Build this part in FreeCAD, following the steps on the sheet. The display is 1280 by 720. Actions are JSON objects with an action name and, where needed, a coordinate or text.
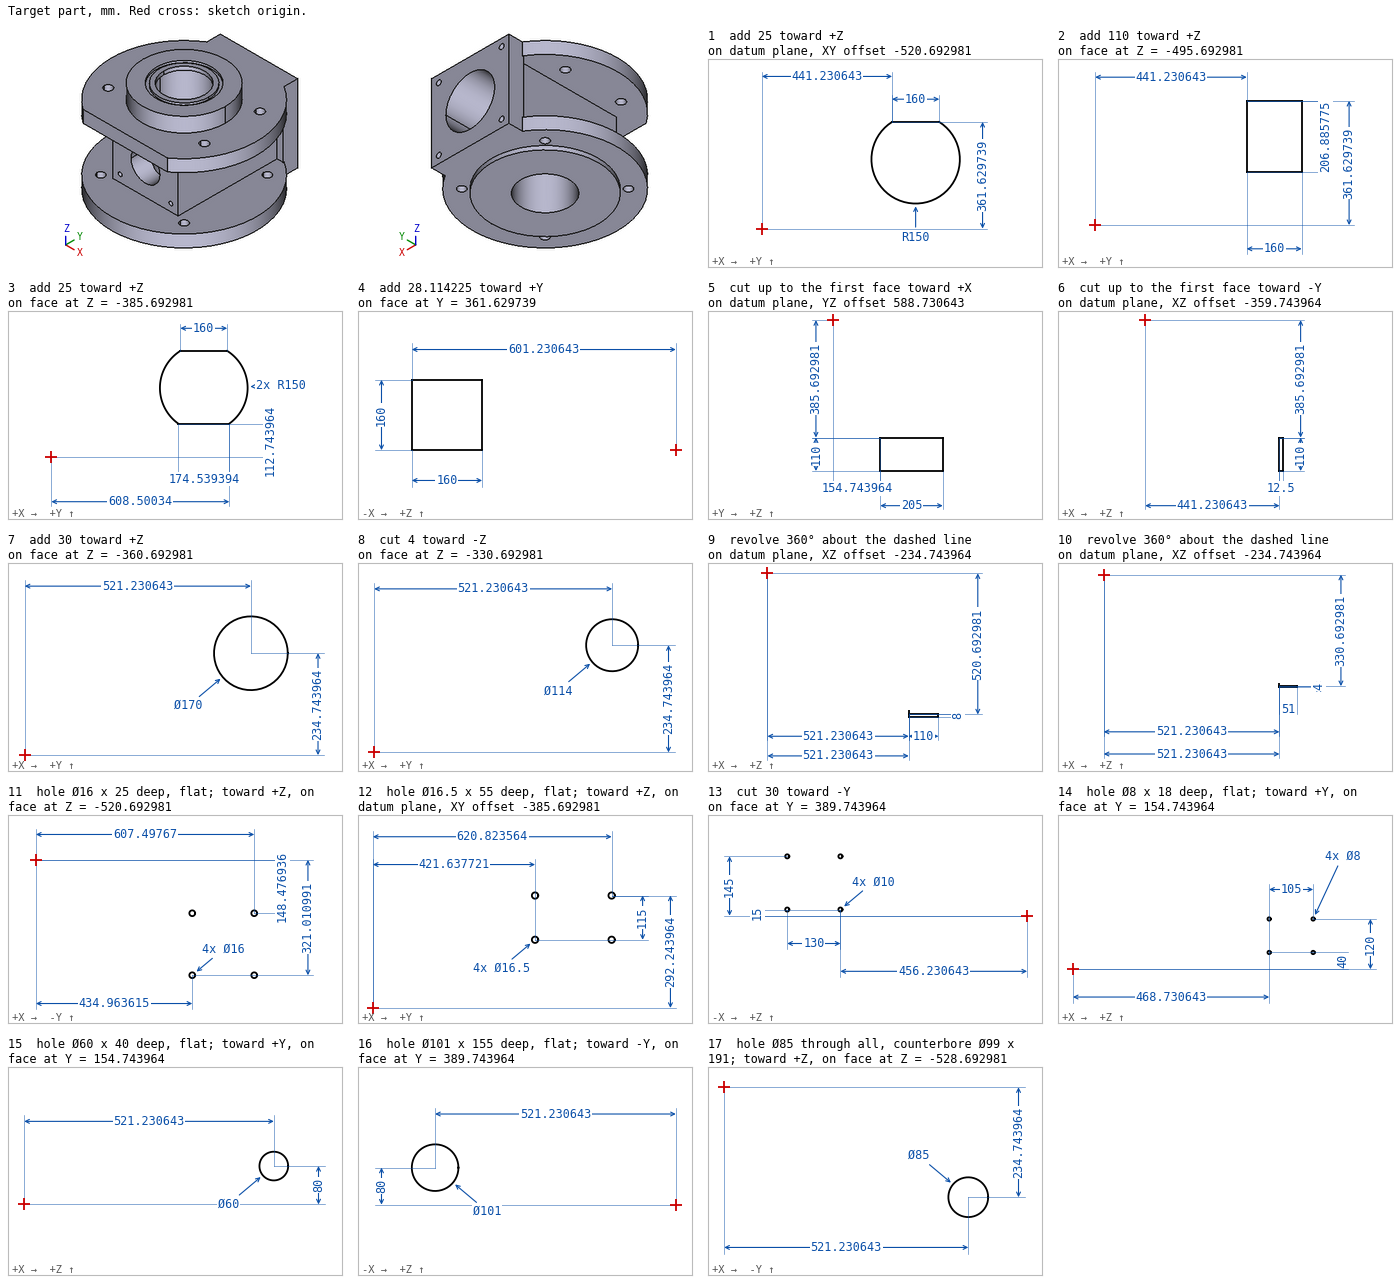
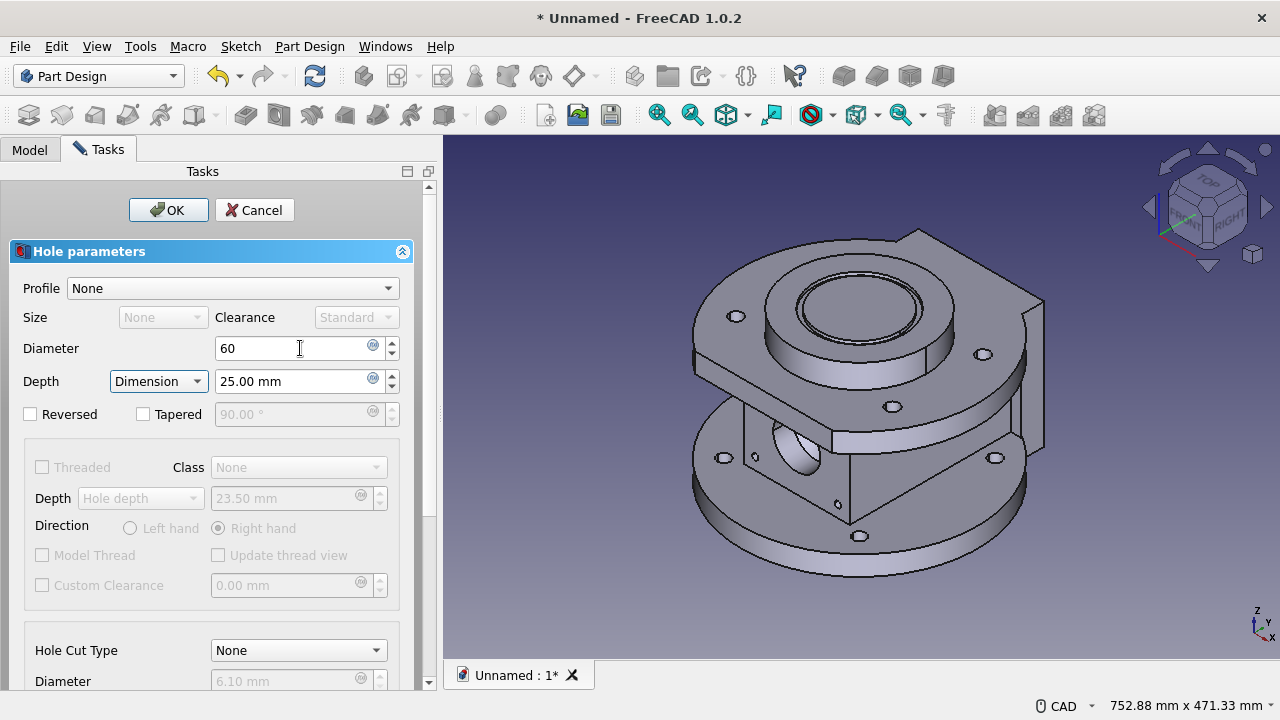
{"action": "triple_click", "coordinate": [300, 382]}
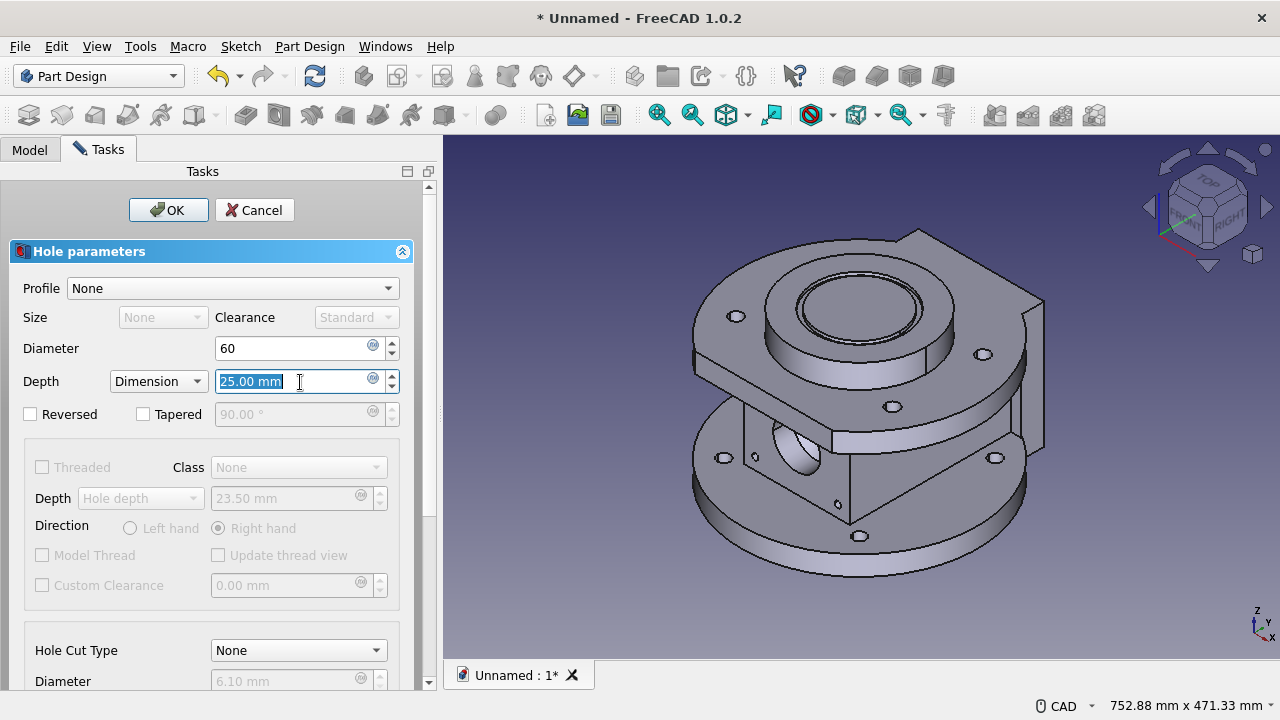
{"action": "type", "text": "40"}
{"action": "key", "text": "Tab"}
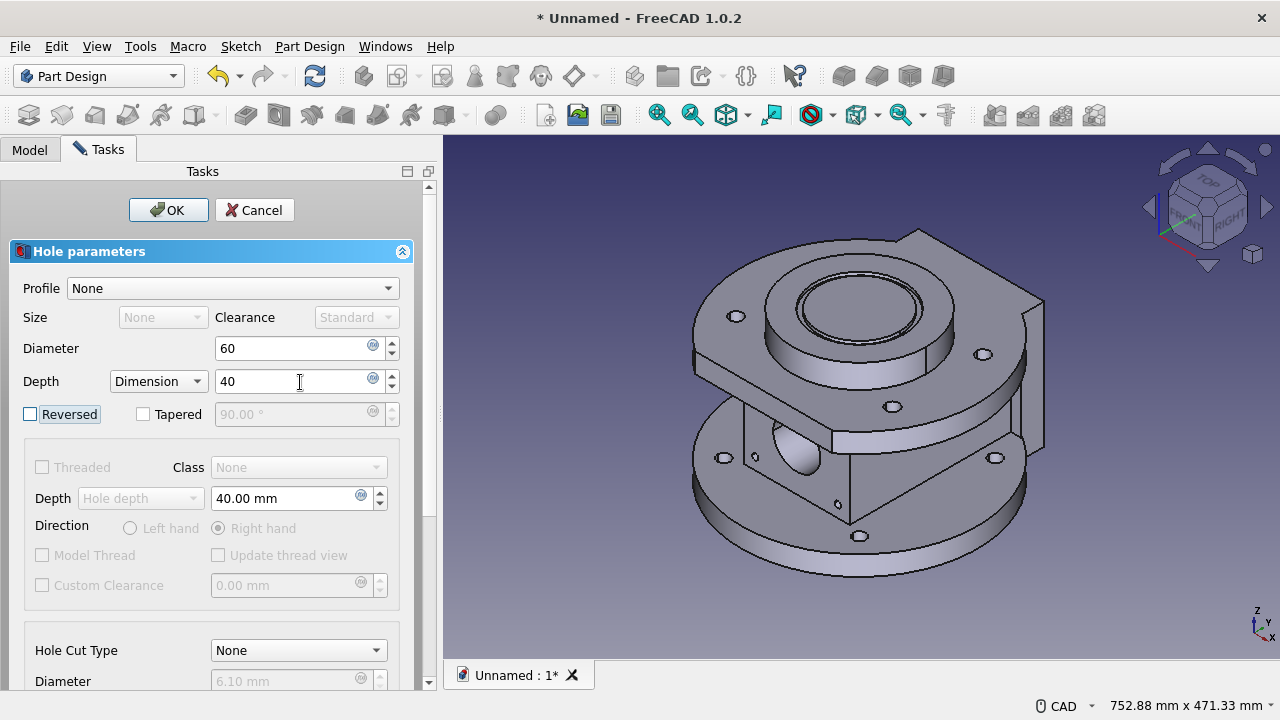
{"action": "scroll", "coordinate": [429, 436], "scroll_direction": "down", "scroll_amount": 4}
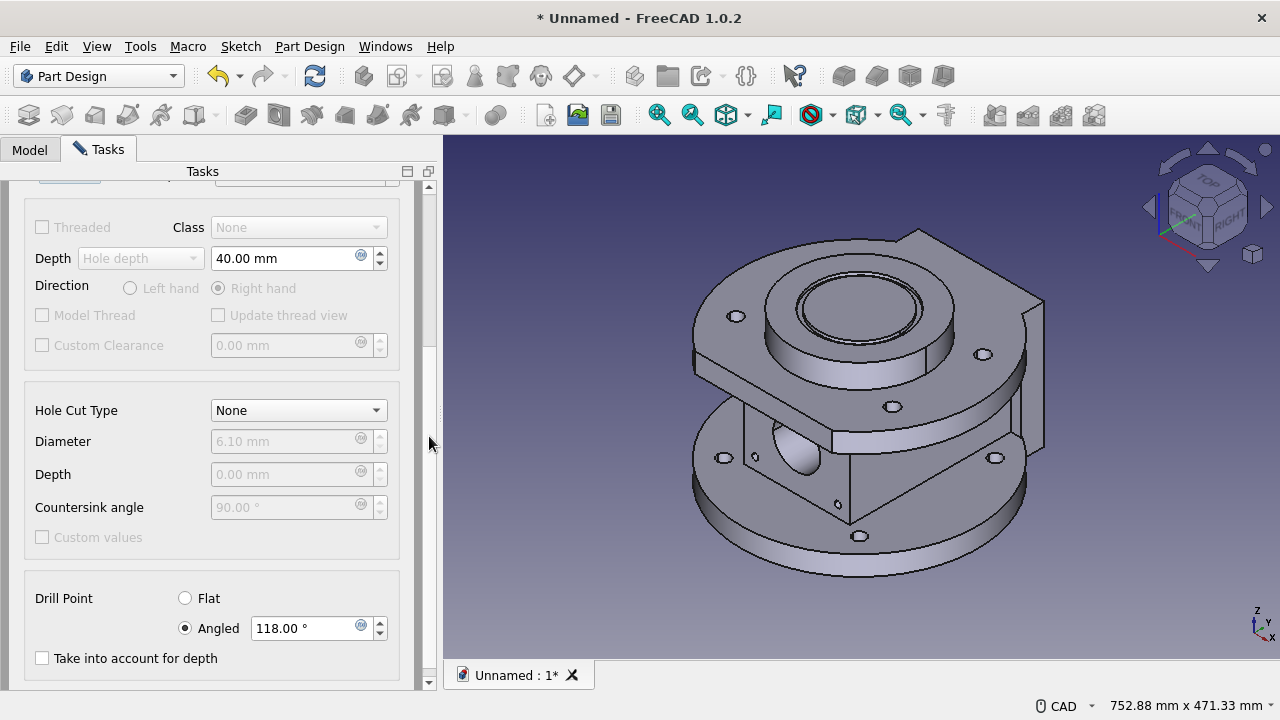
{"action": "left_click", "coordinate": [186, 596]}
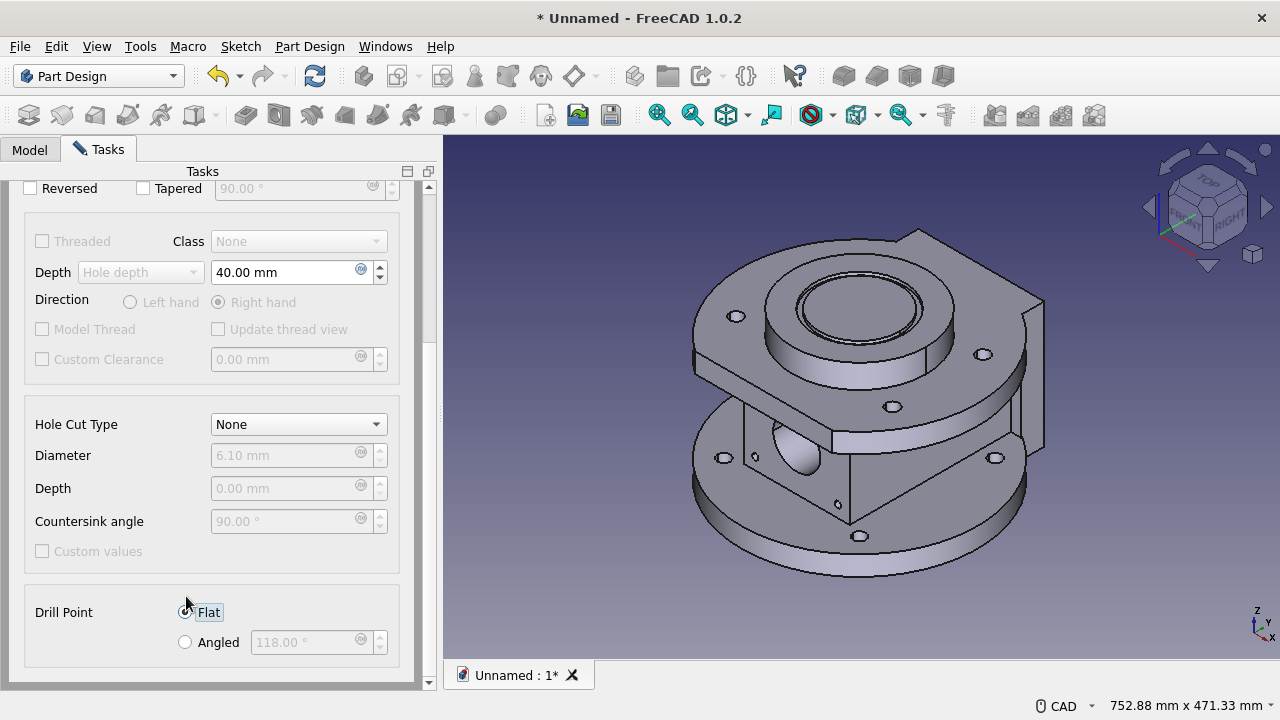
{"action": "scroll", "coordinate": [429, 436], "scroll_direction": "up", "scroll_amount": 5}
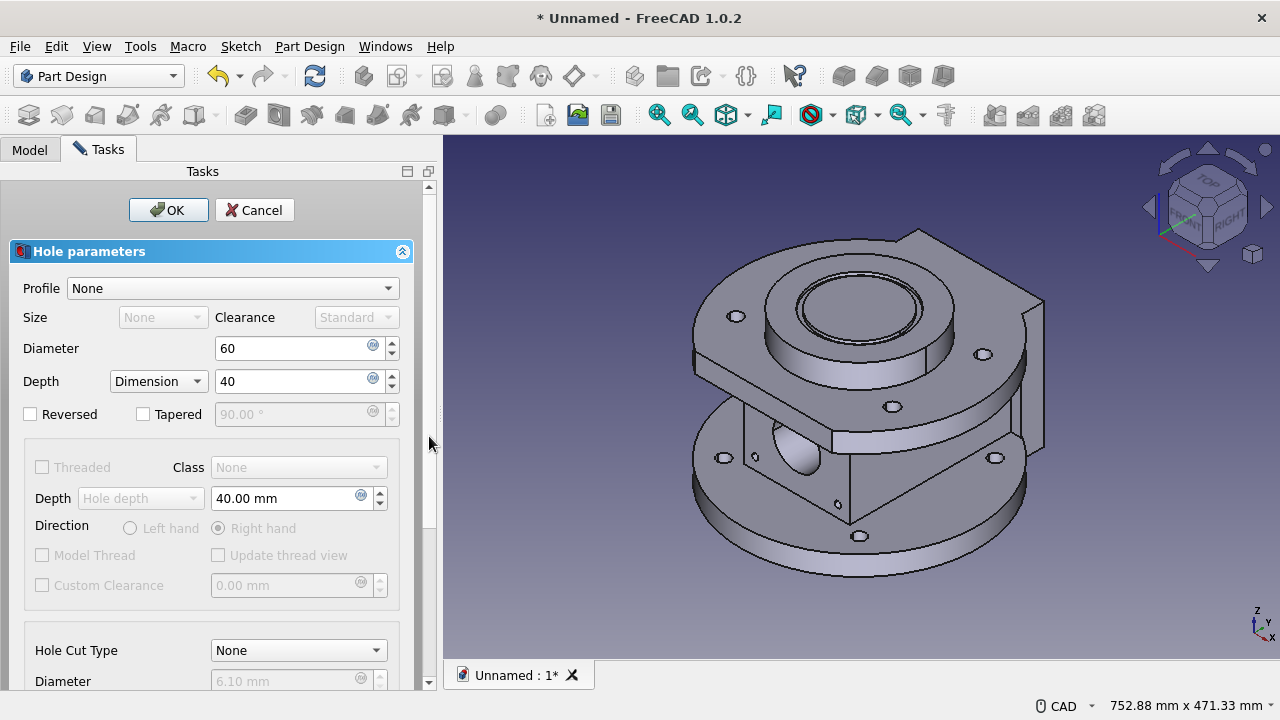
{"action": "left_click", "coordinate": [169, 210]}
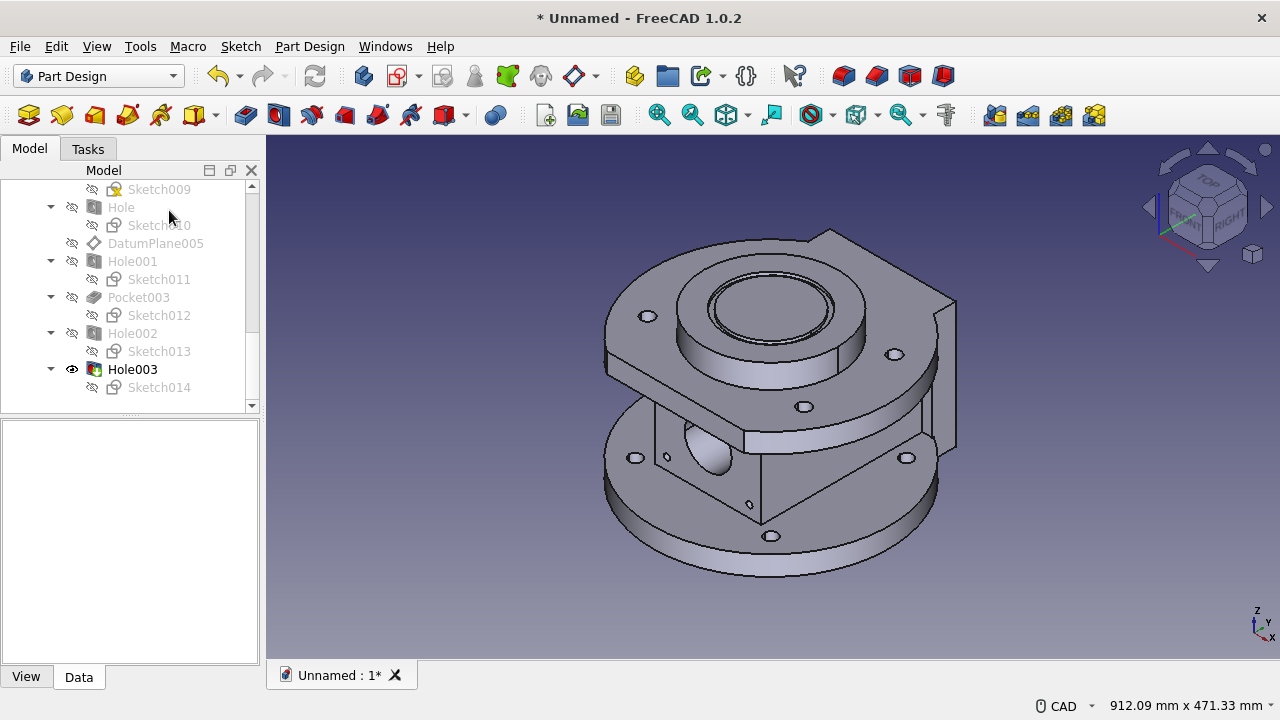
{"action": "key", "text": "4"}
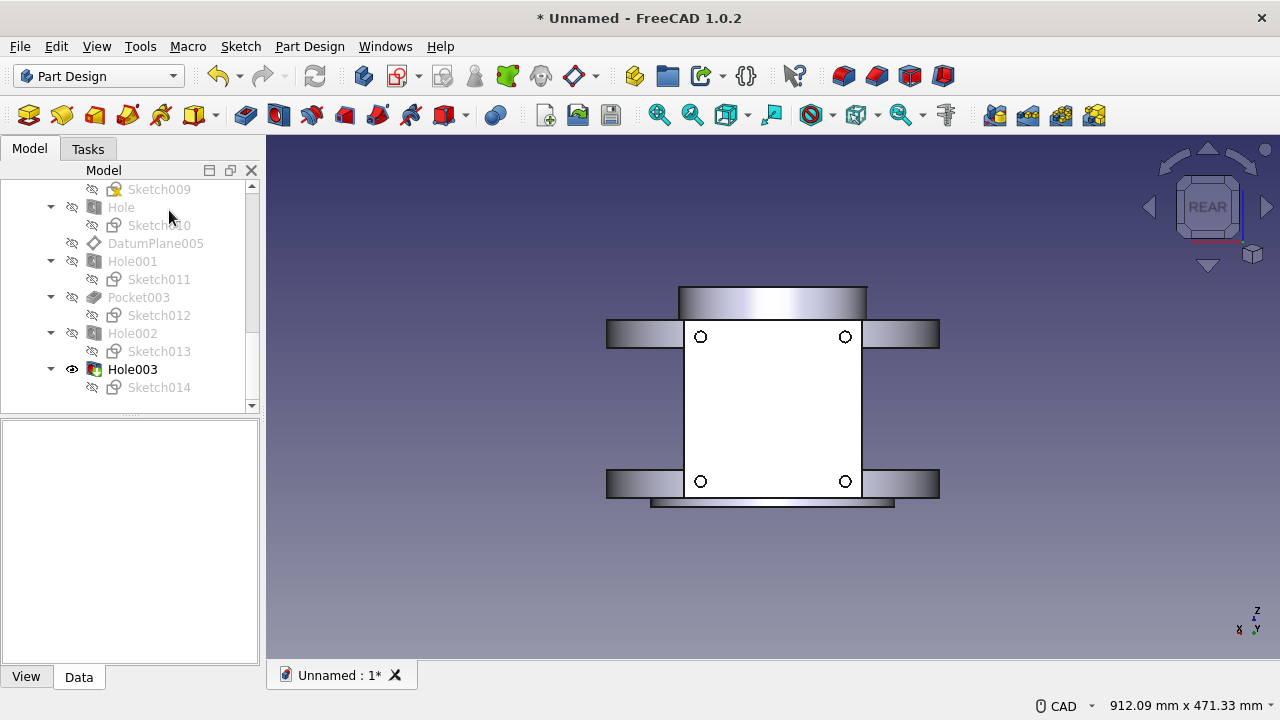
{"action": "left_click", "coordinate": [660, 116]}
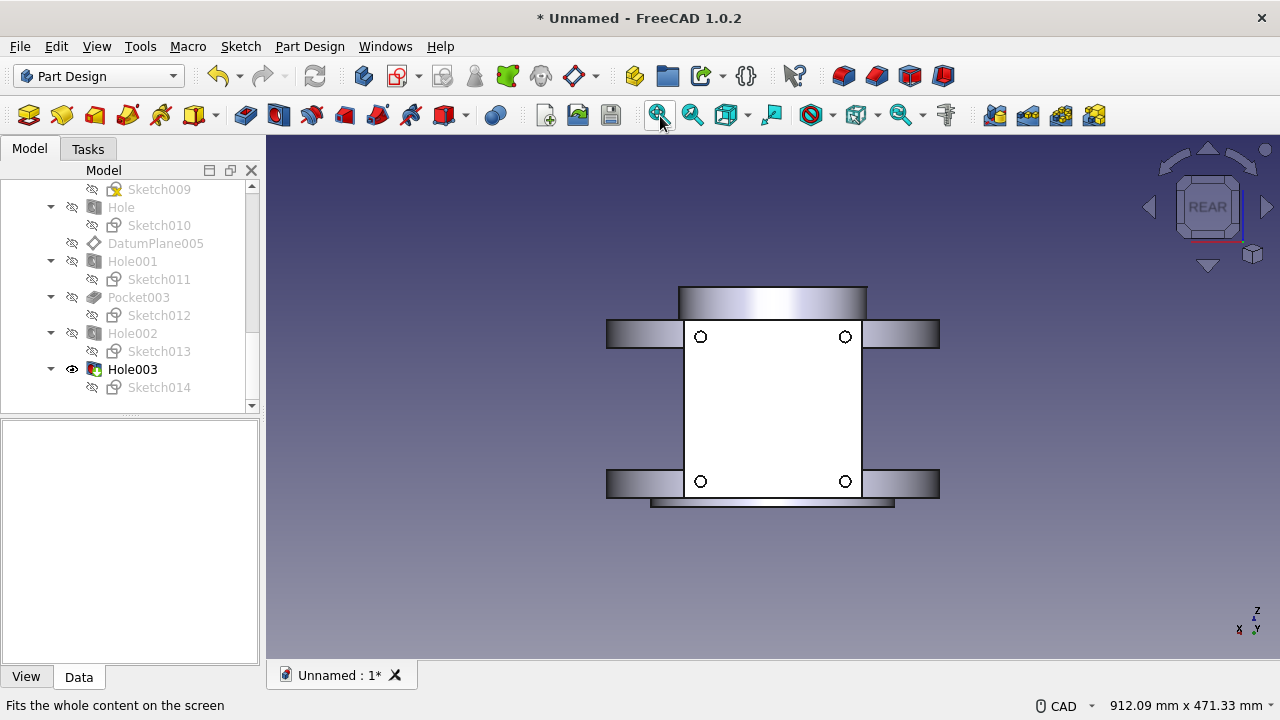
{"action": "left_click", "coordinate": [773, 408]}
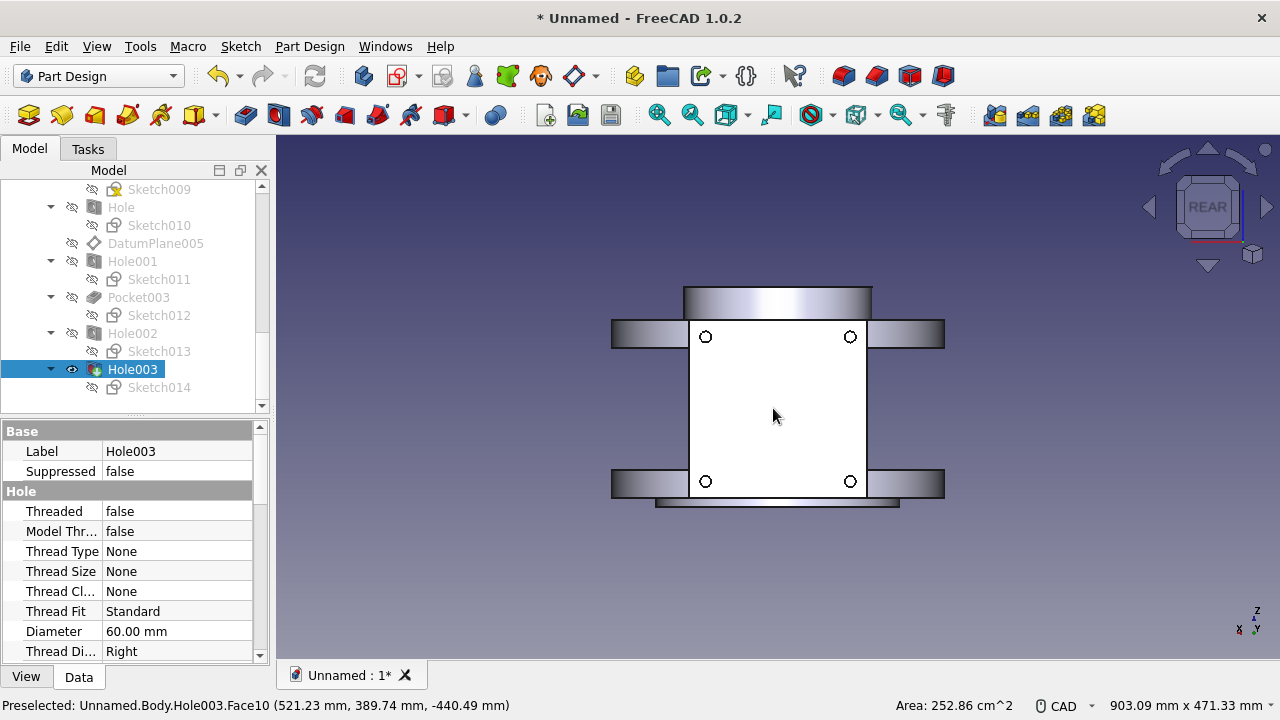
{"action": "left_click", "coordinate": [396, 76]}